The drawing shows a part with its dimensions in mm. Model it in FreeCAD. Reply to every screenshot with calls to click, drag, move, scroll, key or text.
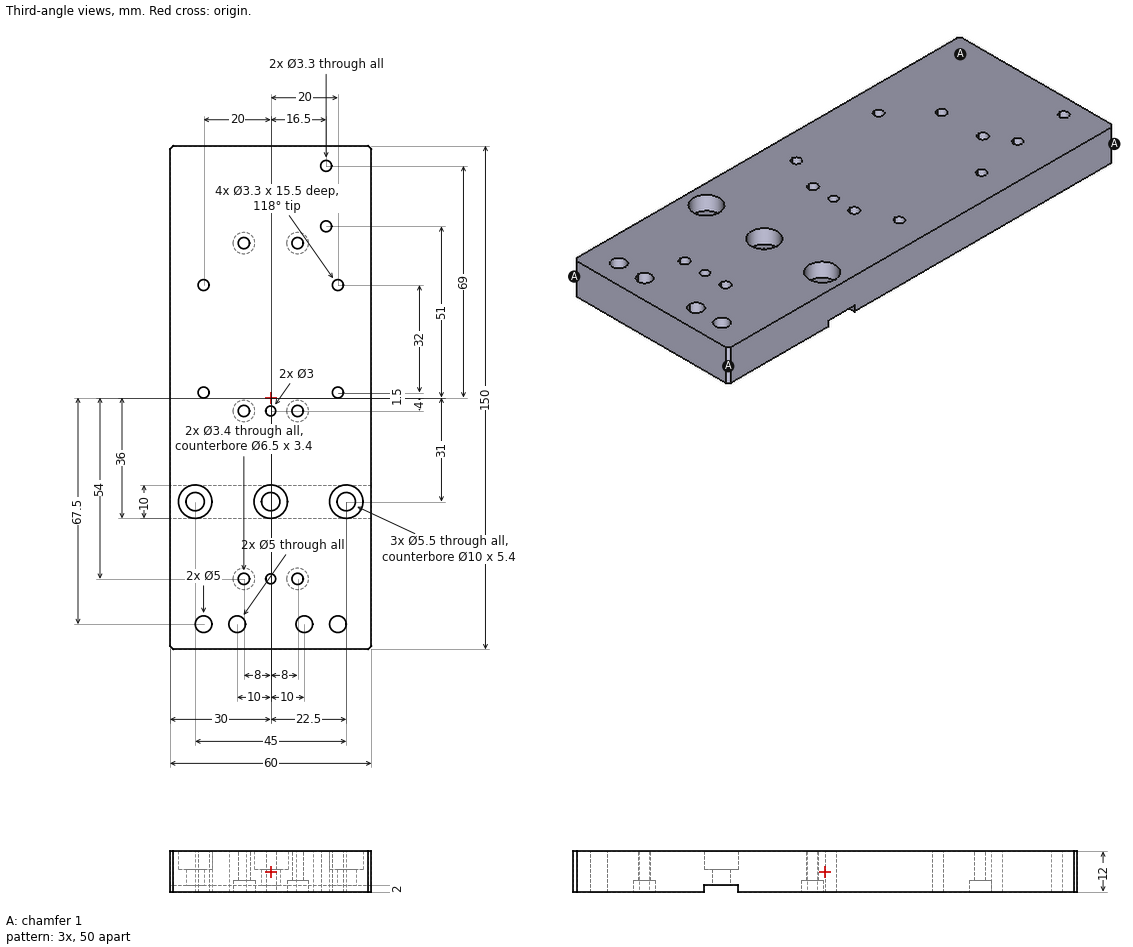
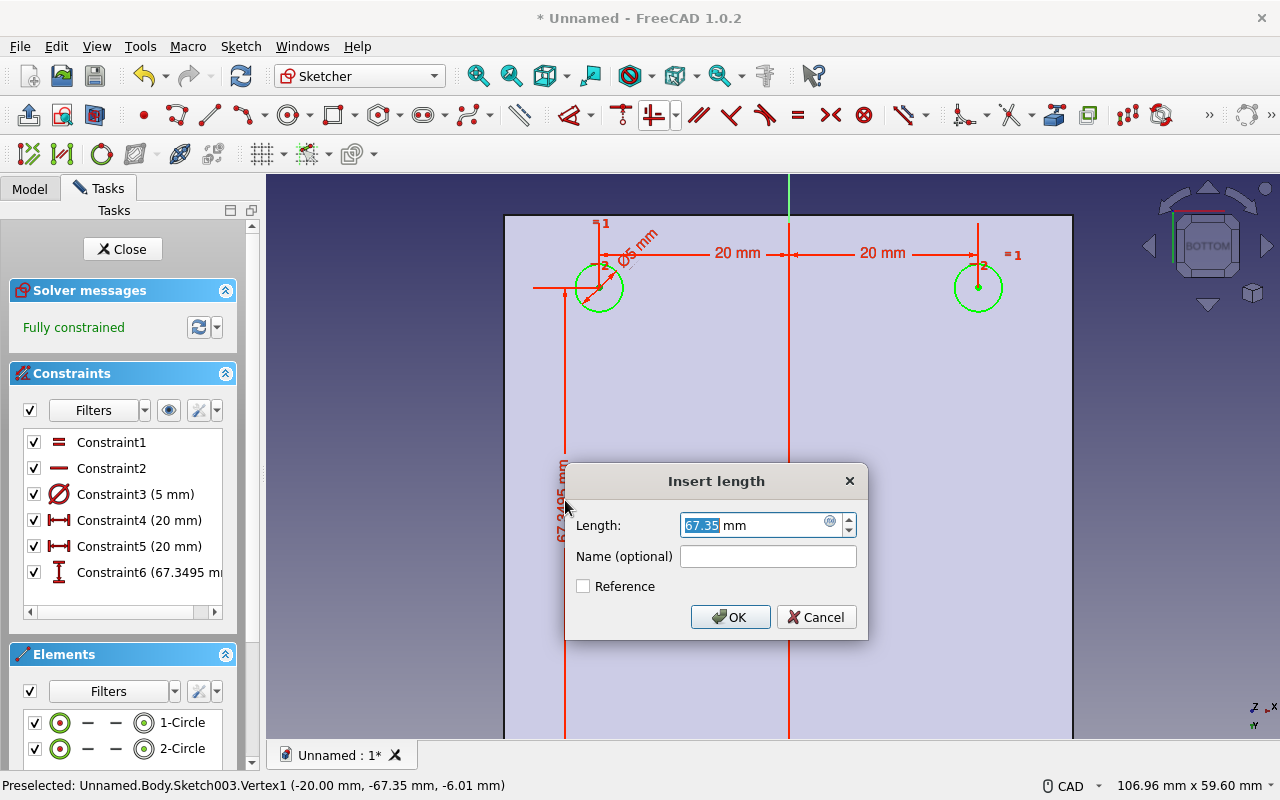
text(67.5)
key(Return)
key(Escape)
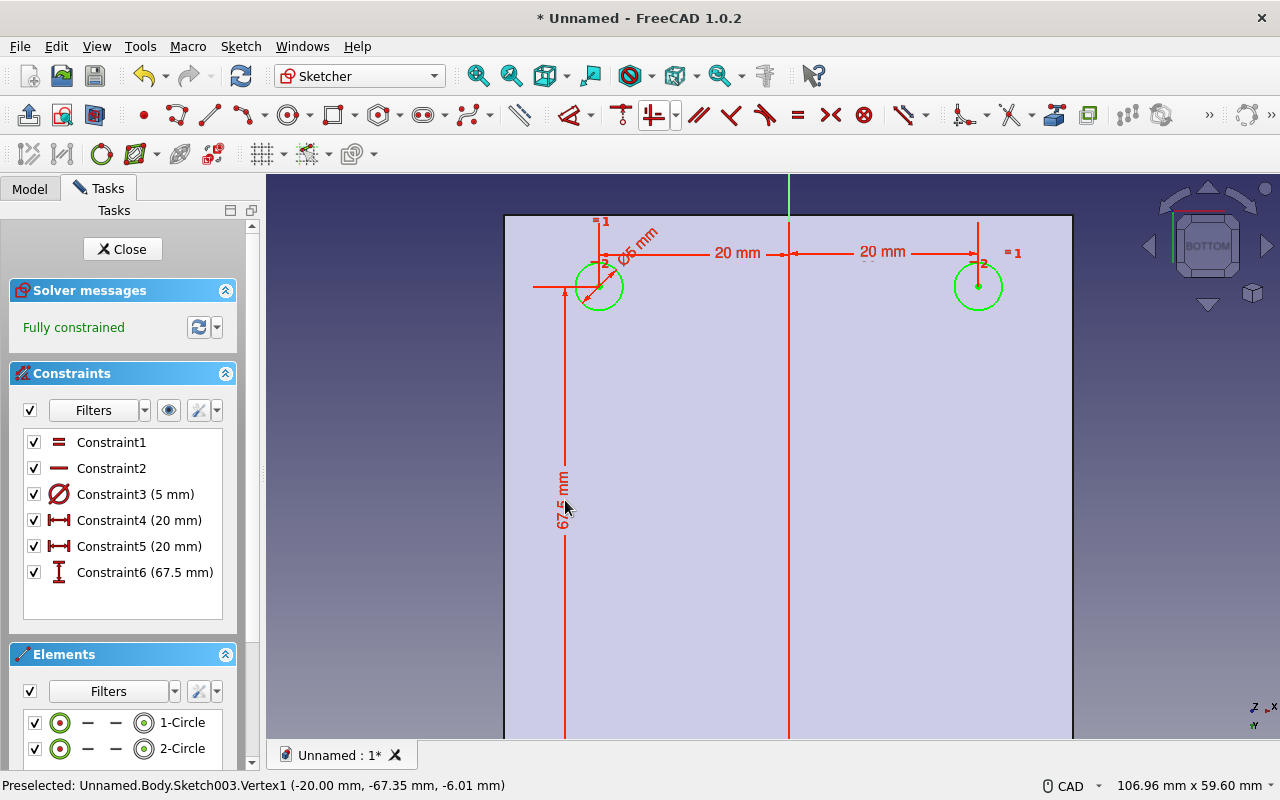
click(123, 249)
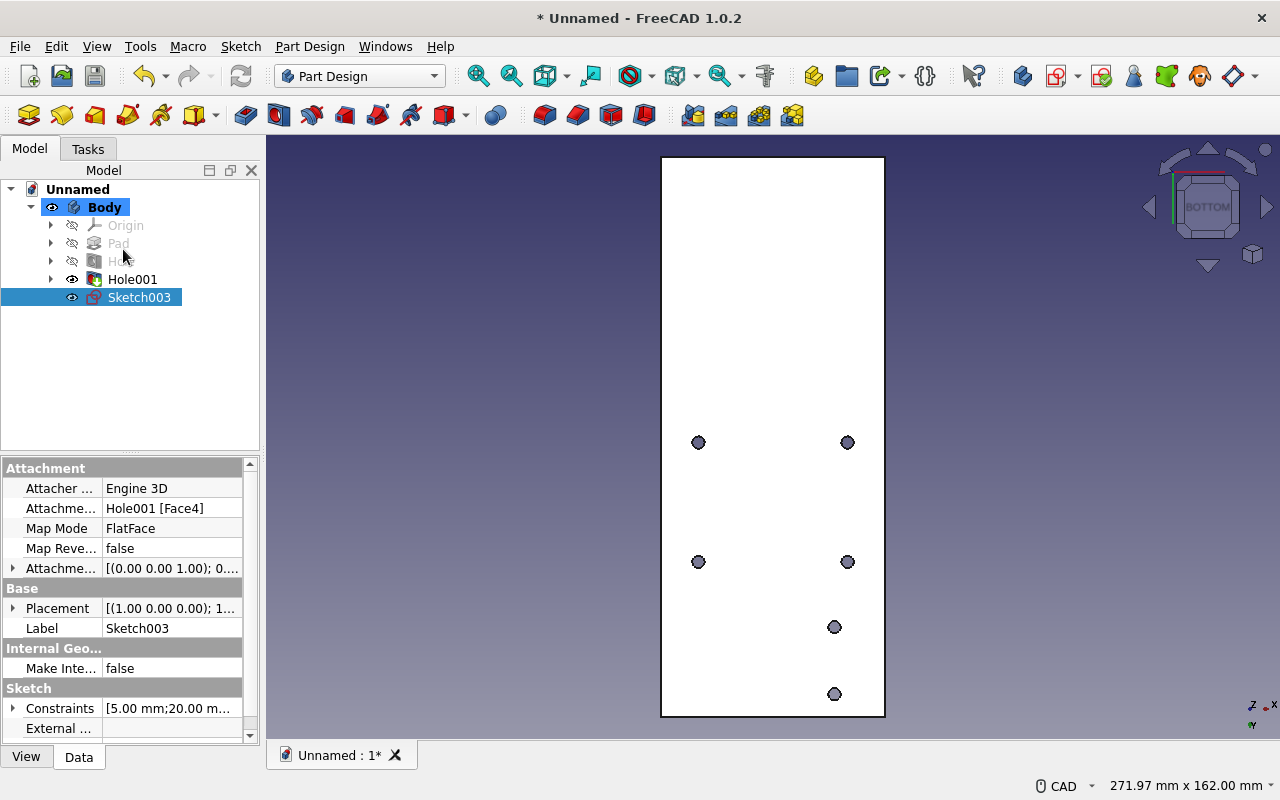
click(246, 116)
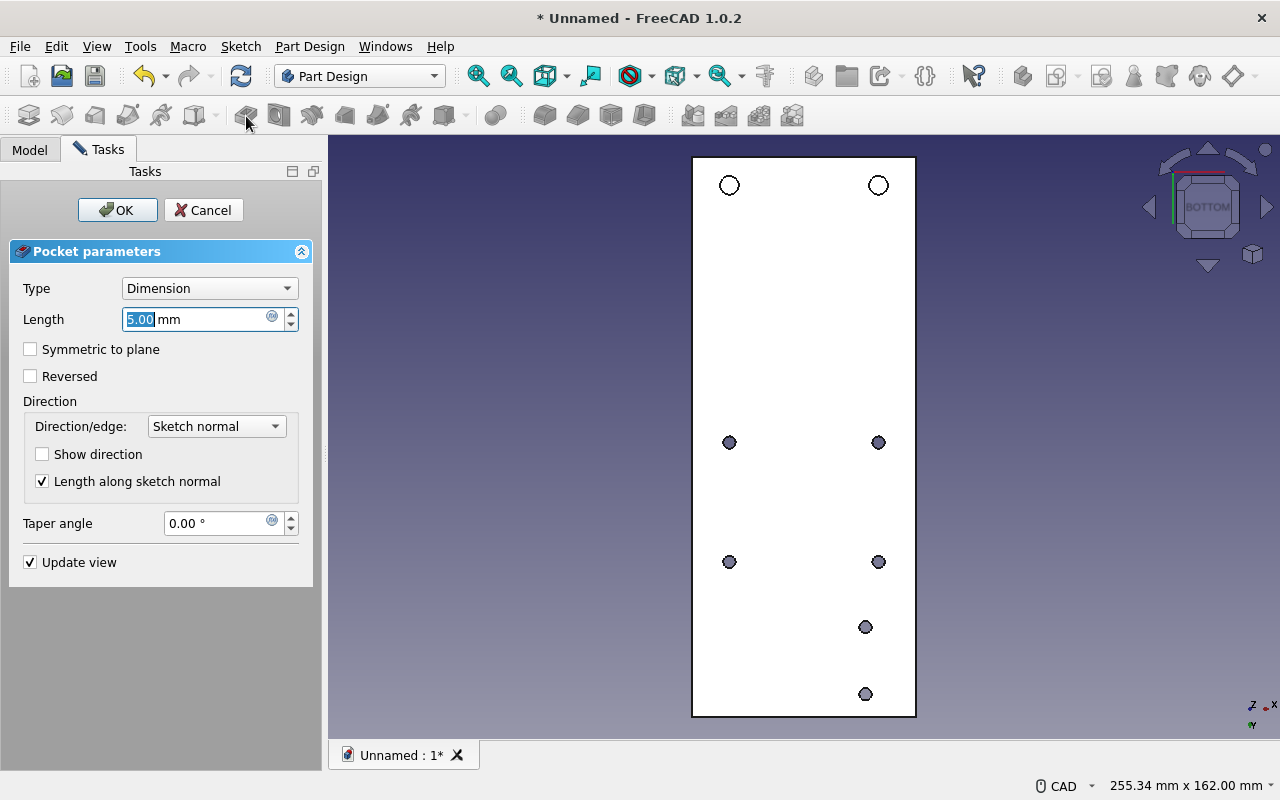
click(210, 288)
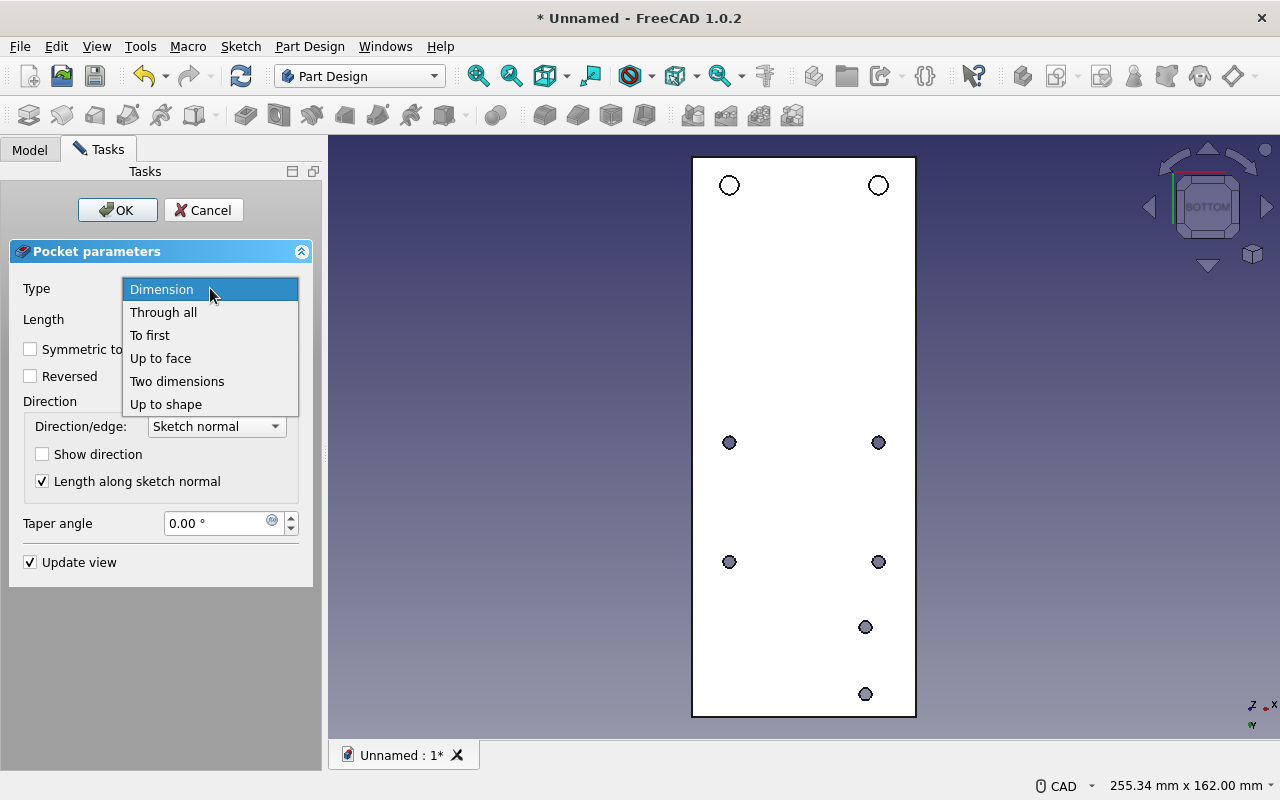
click(208, 312)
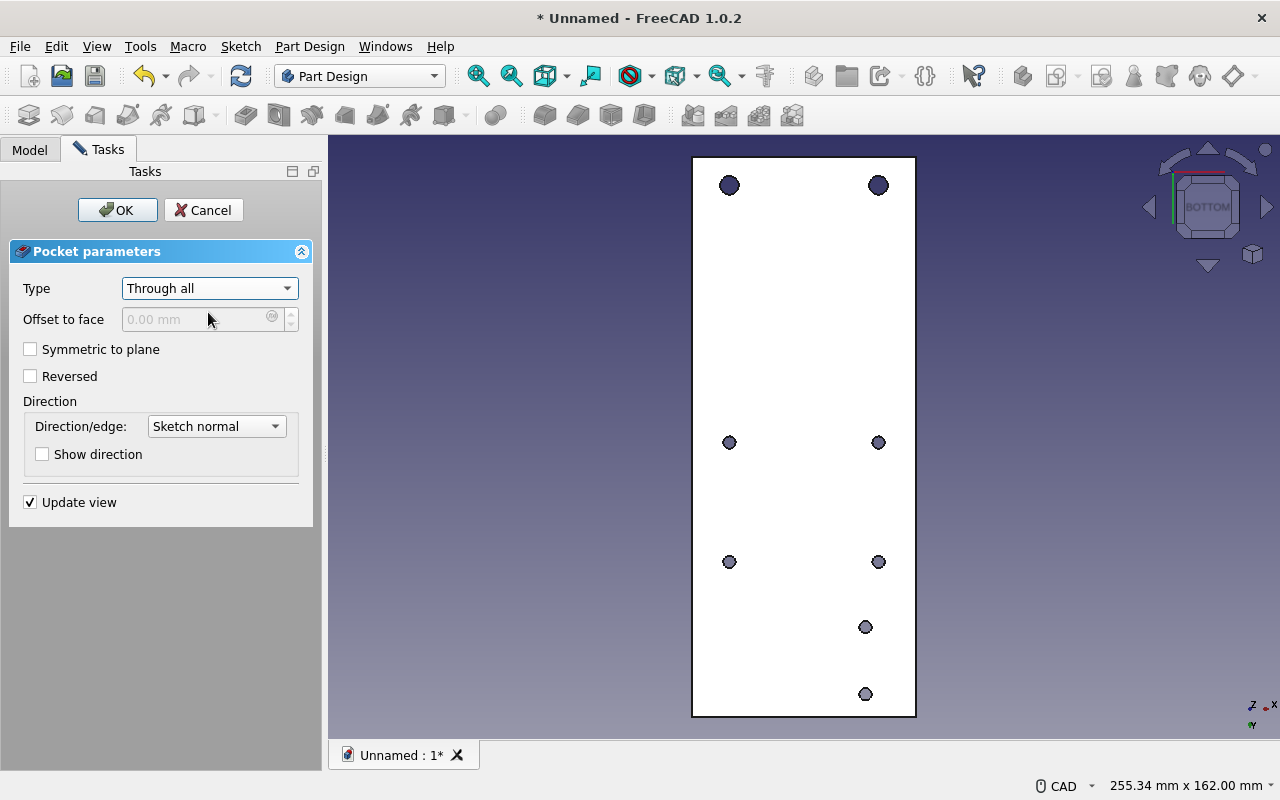
click(118, 210)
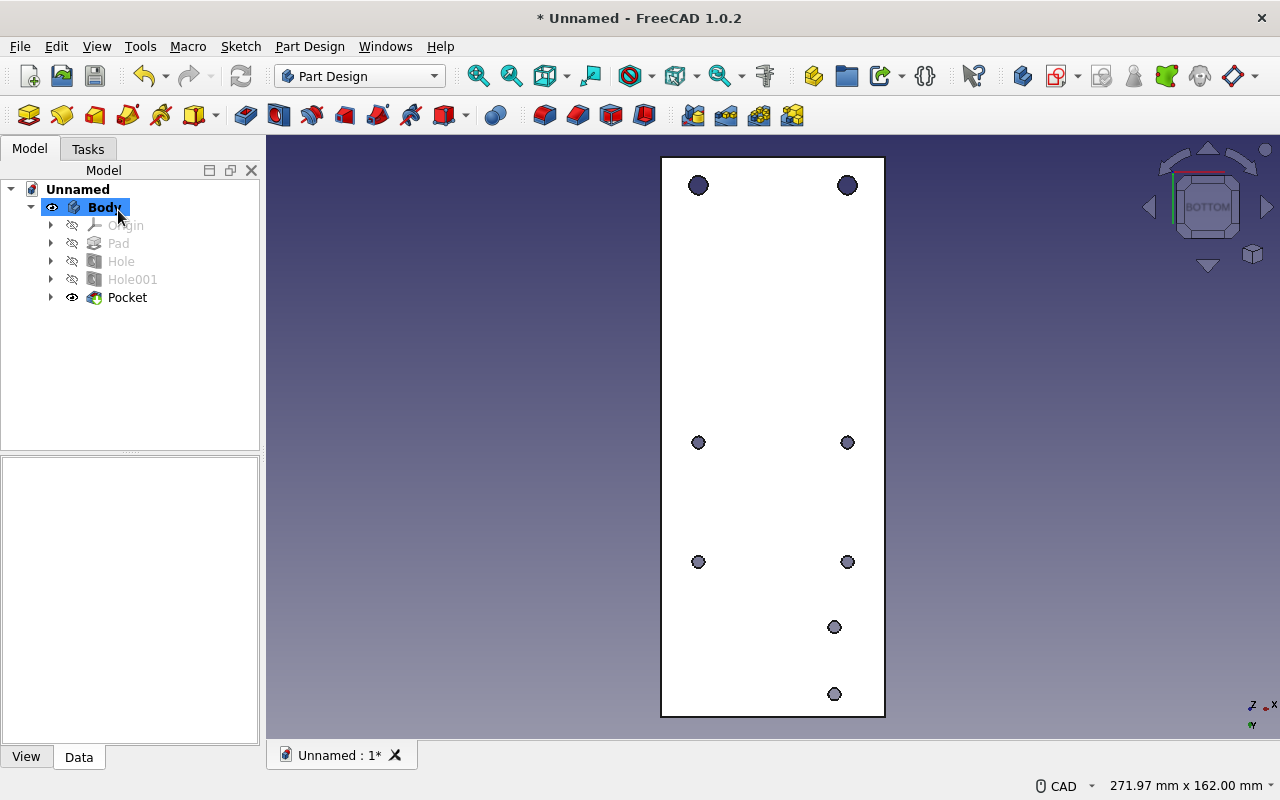
click(773, 276)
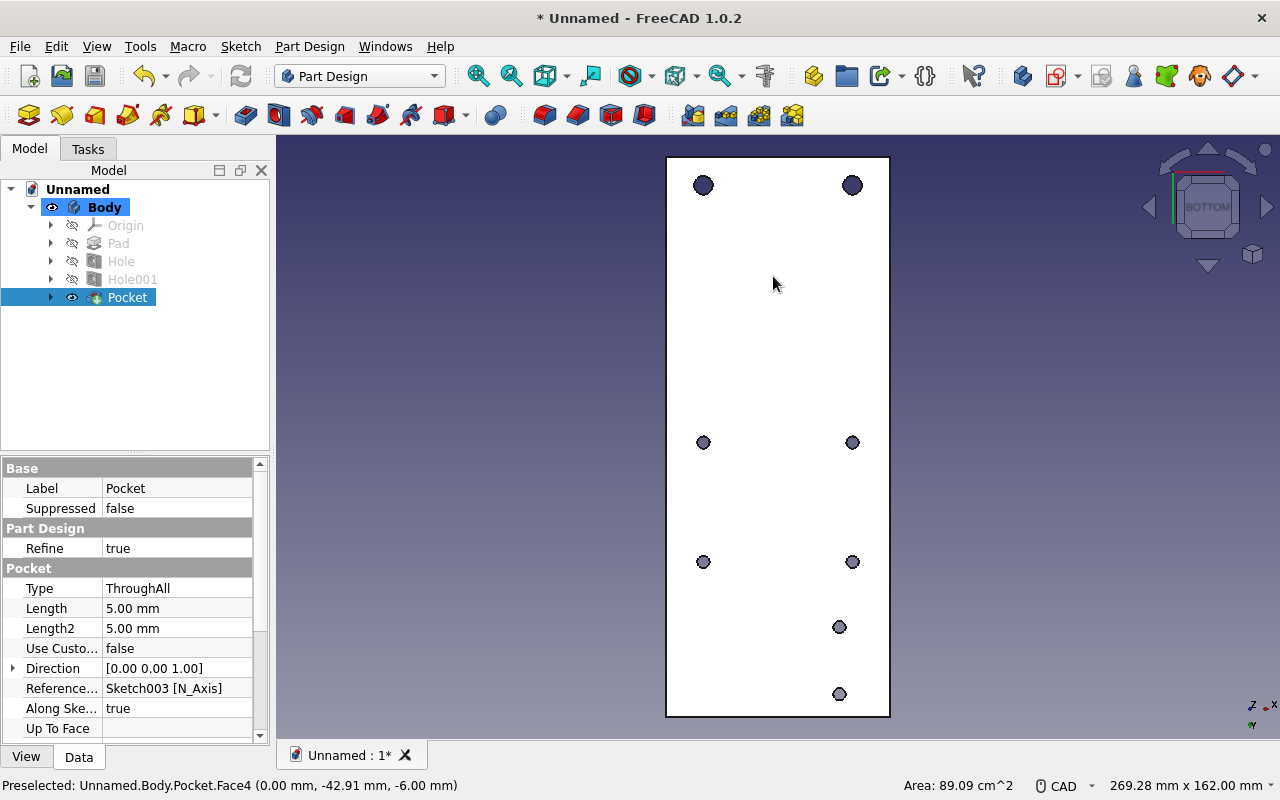
click(1056, 76)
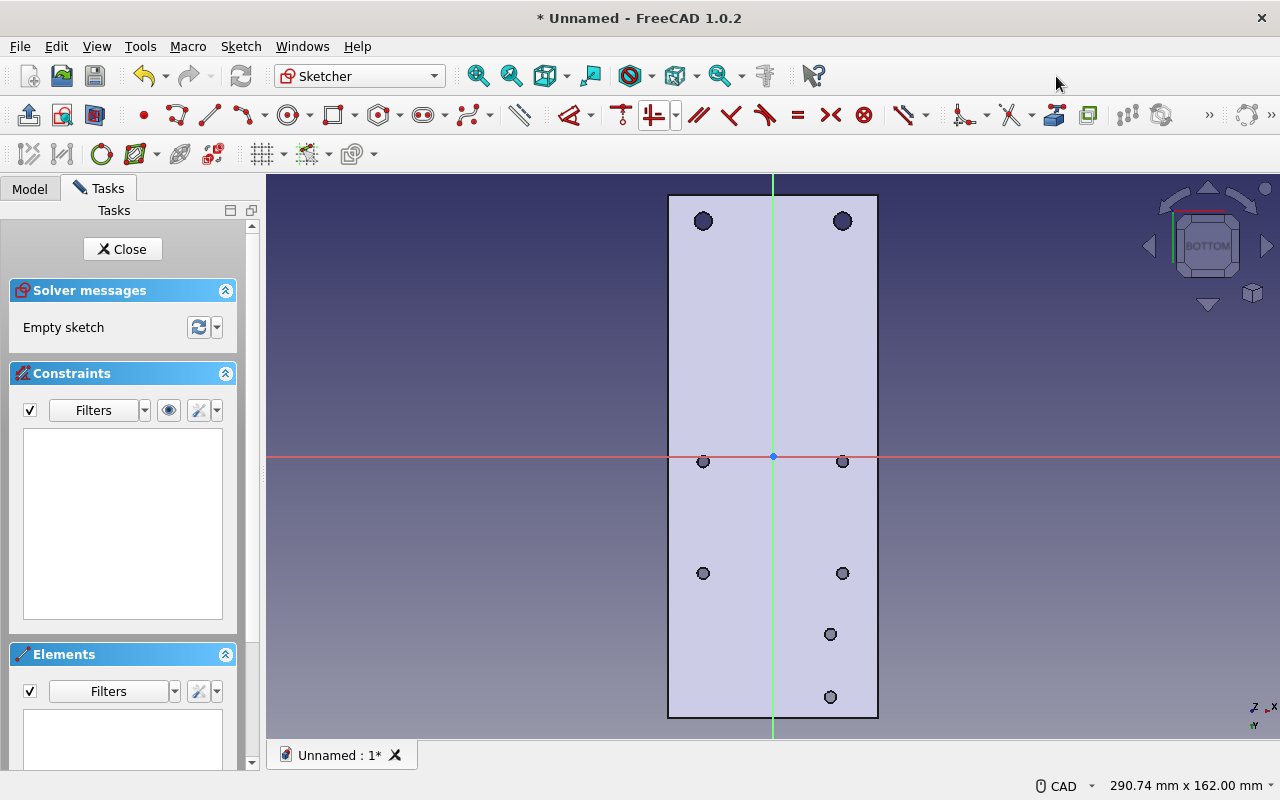
scroll(787, 202, up, 9)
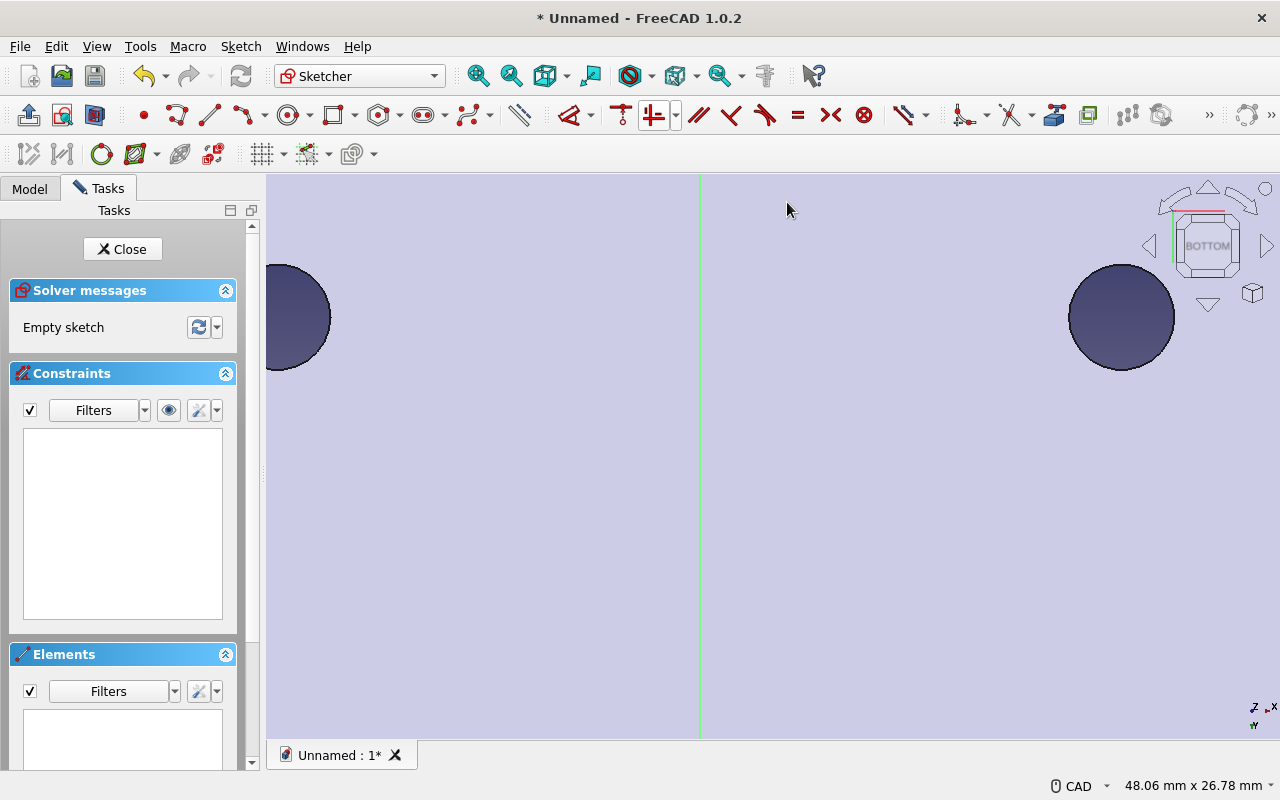
click(288, 116)